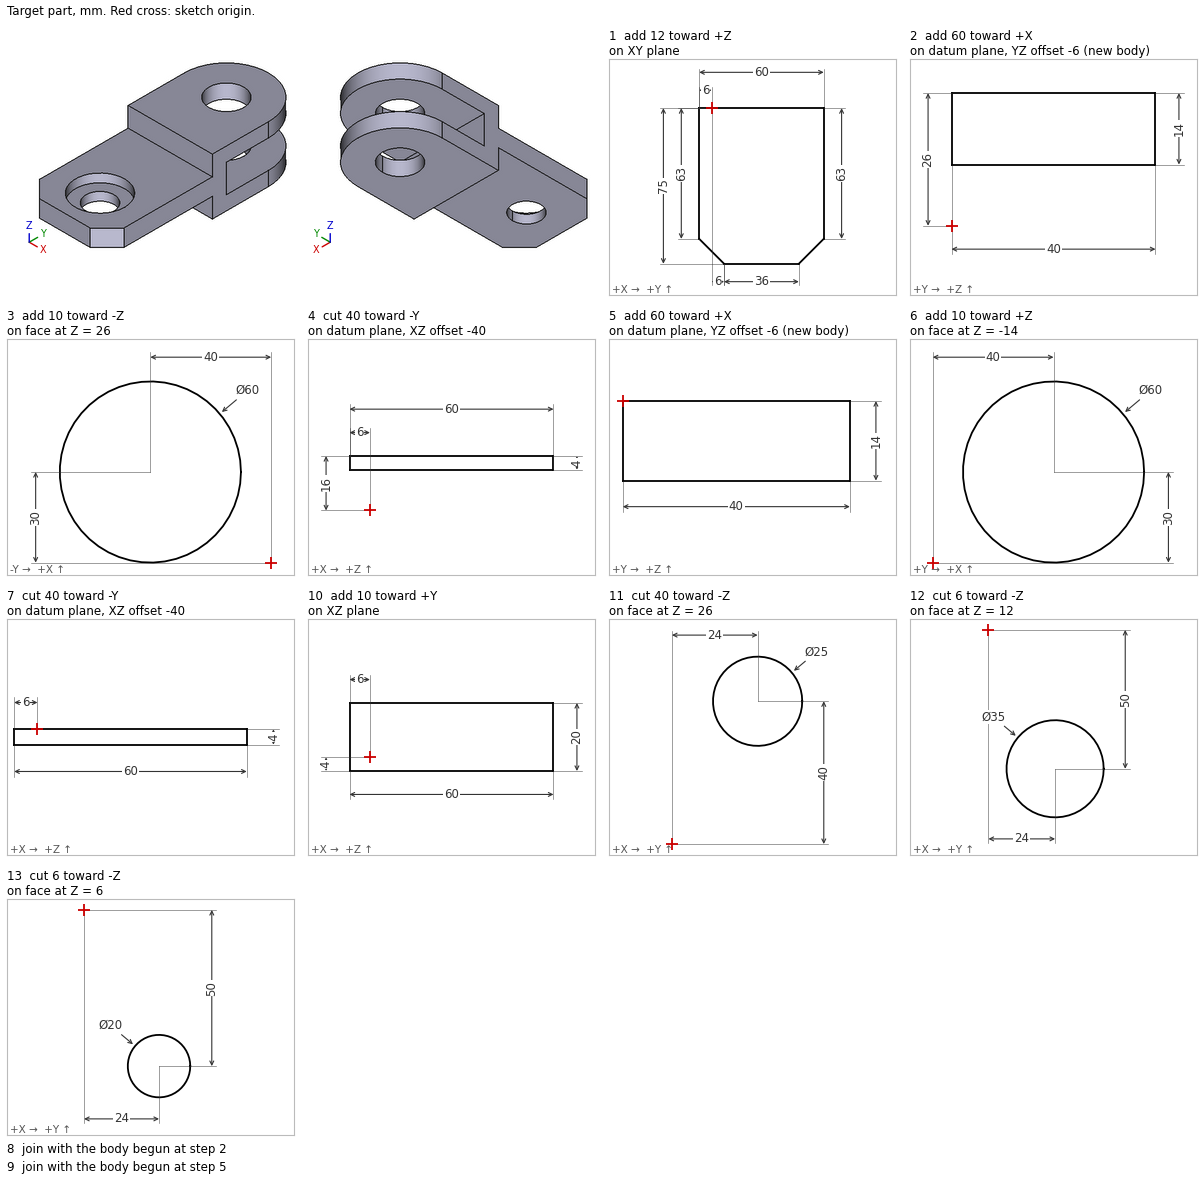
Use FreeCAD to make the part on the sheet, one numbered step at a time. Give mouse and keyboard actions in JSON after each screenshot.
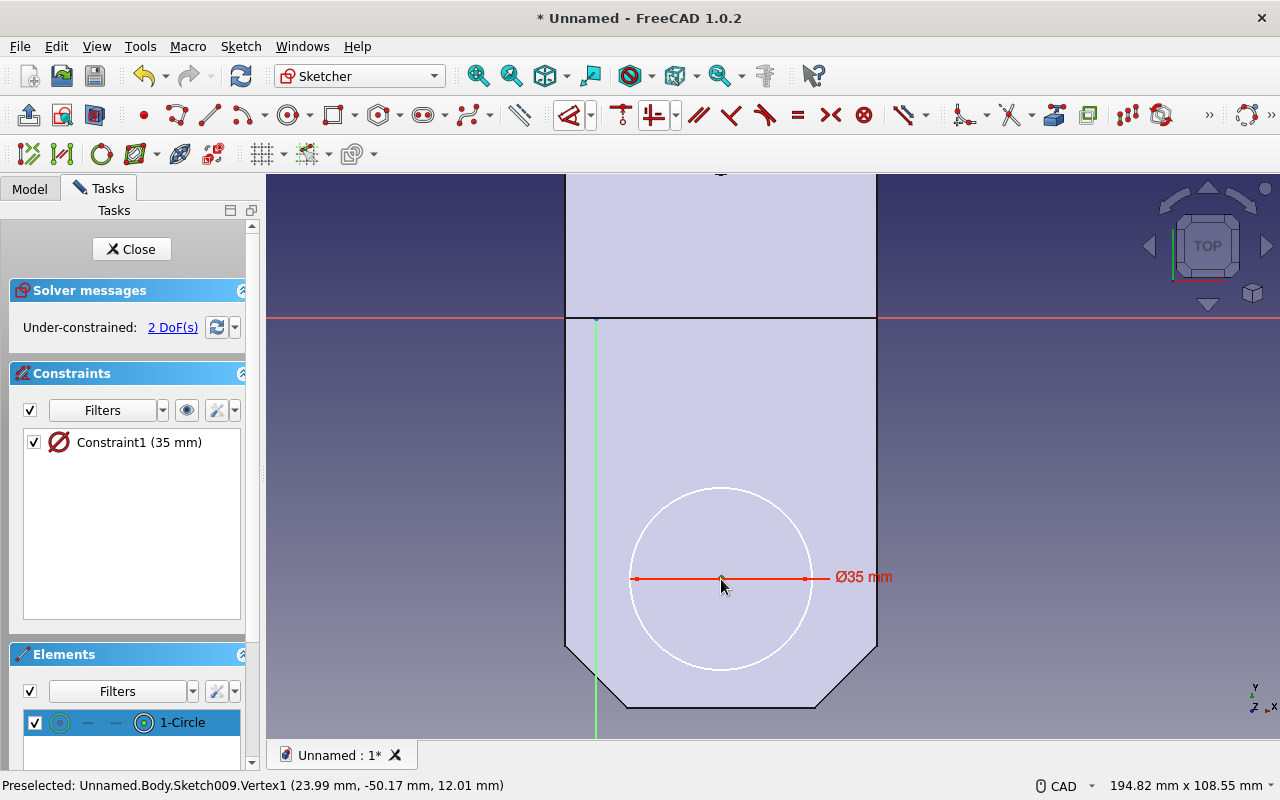
{"action": "left_click", "coordinate": [590, 116]}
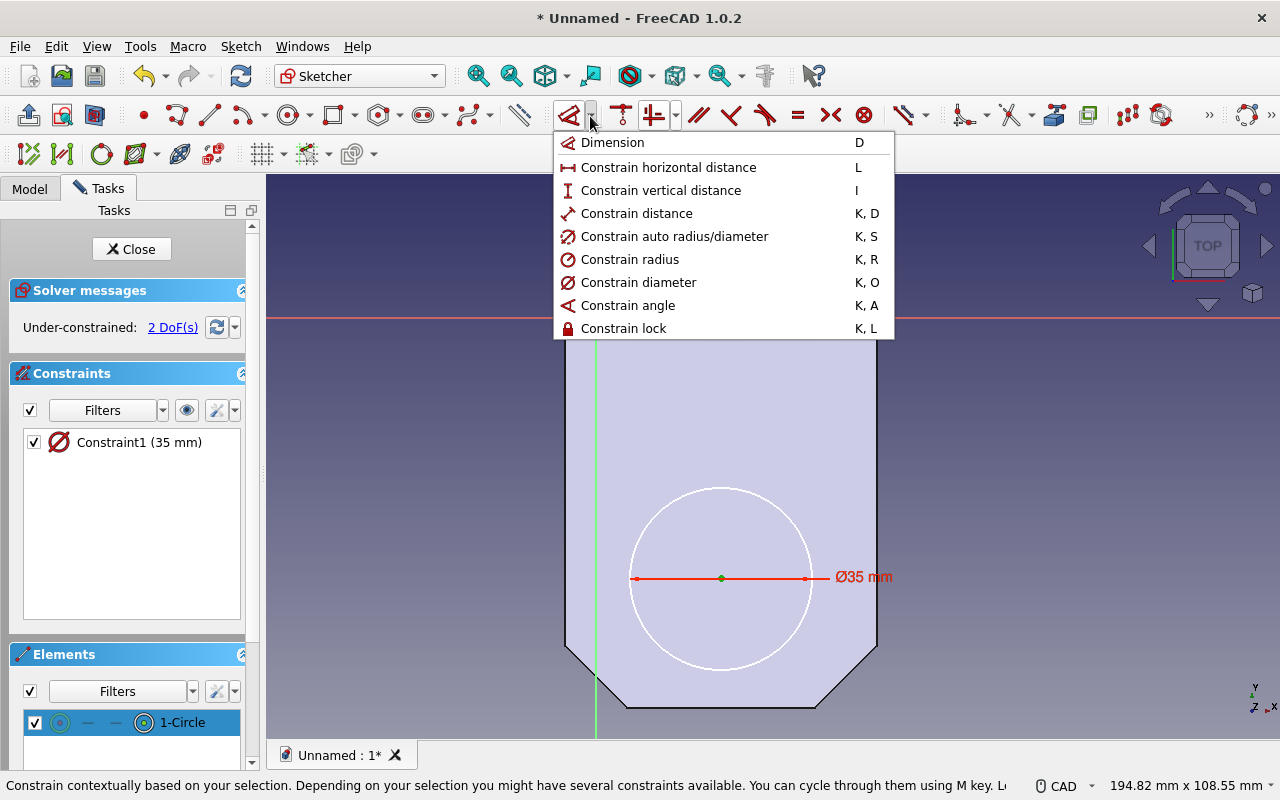
{"action": "left_click", "coordinate": [724, 168]}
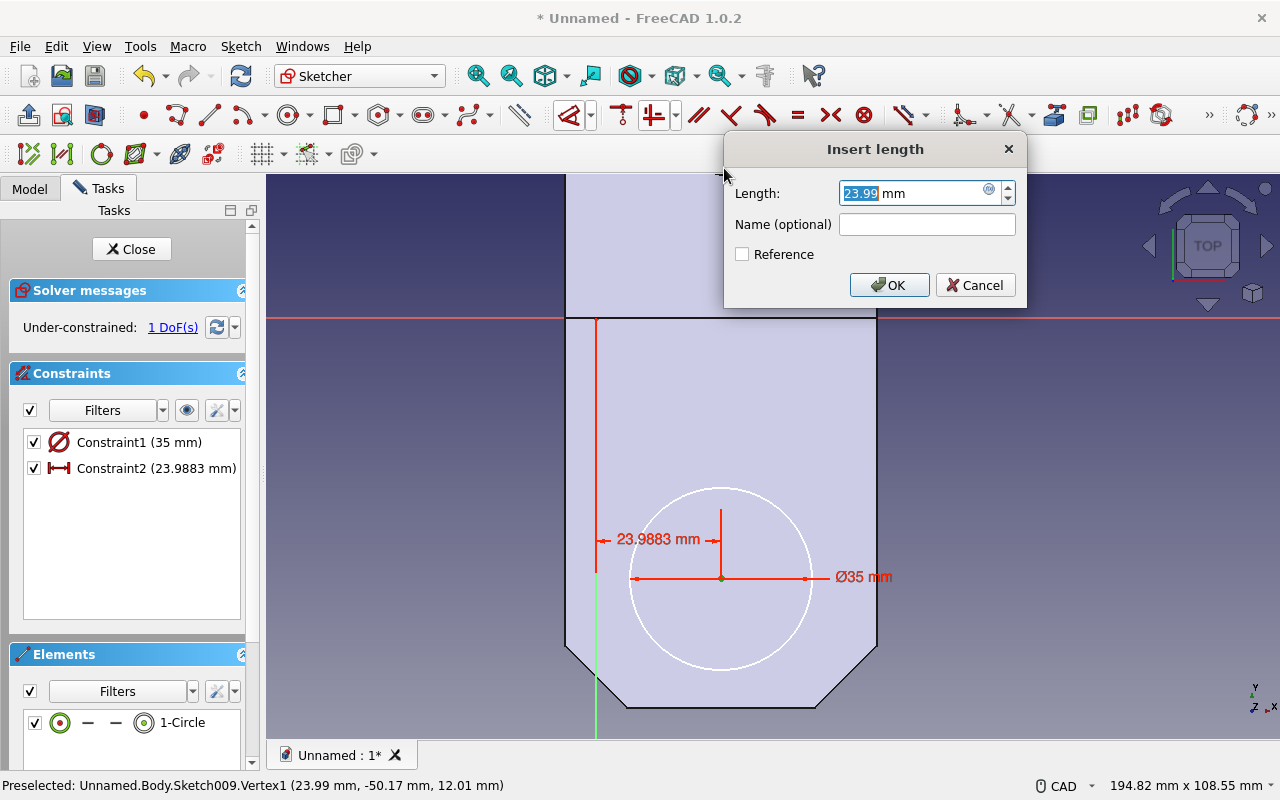
{"action": "type", "text": "24"}
{"action": "key", "text": "Return"}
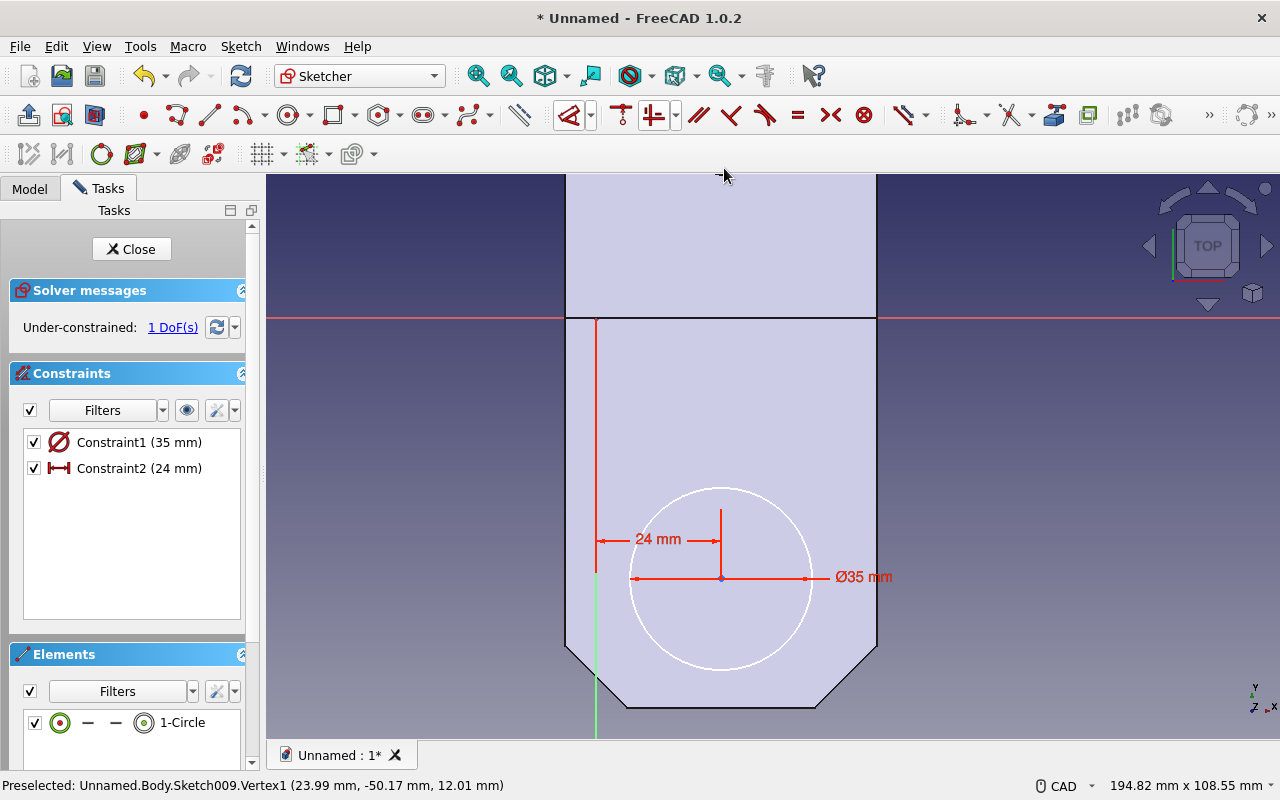
{"action": "left_click", "coordinate": [721, 579]}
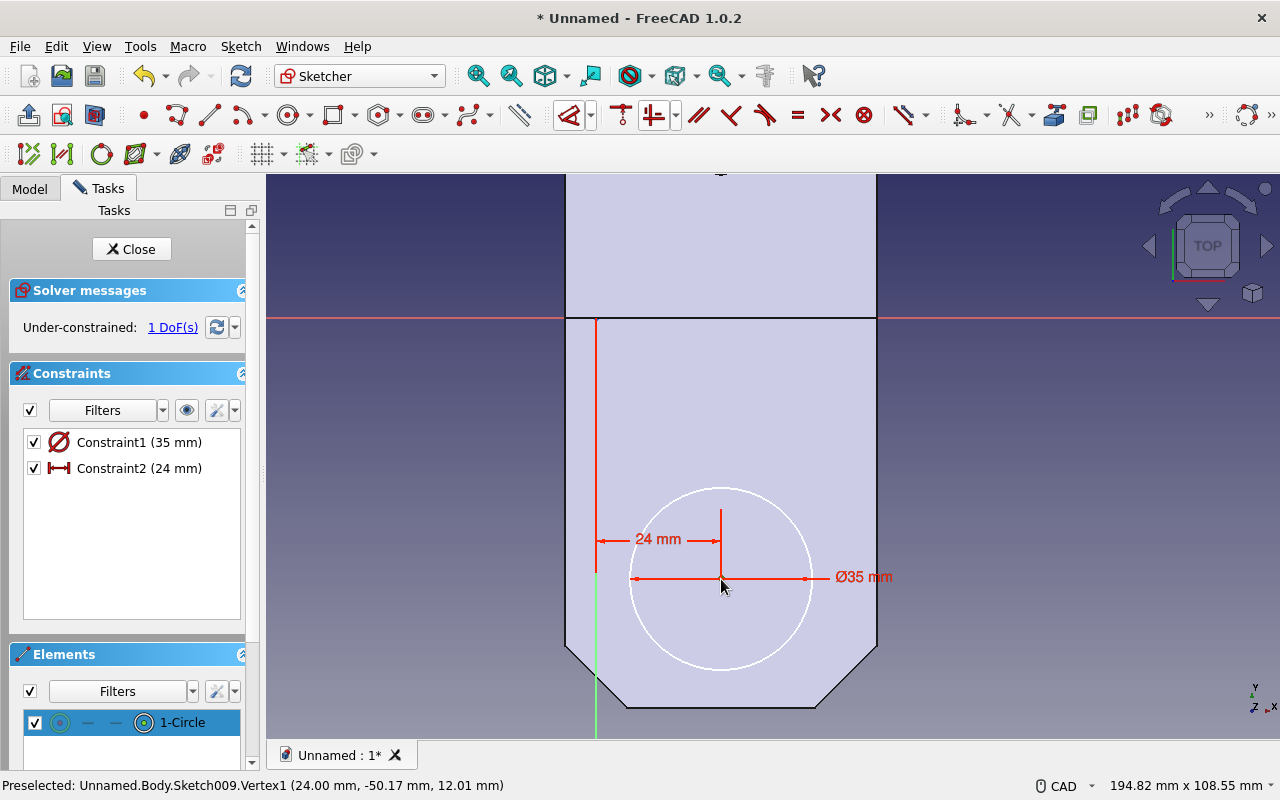
{"action": "left_click", "coordinate": [590, 116]}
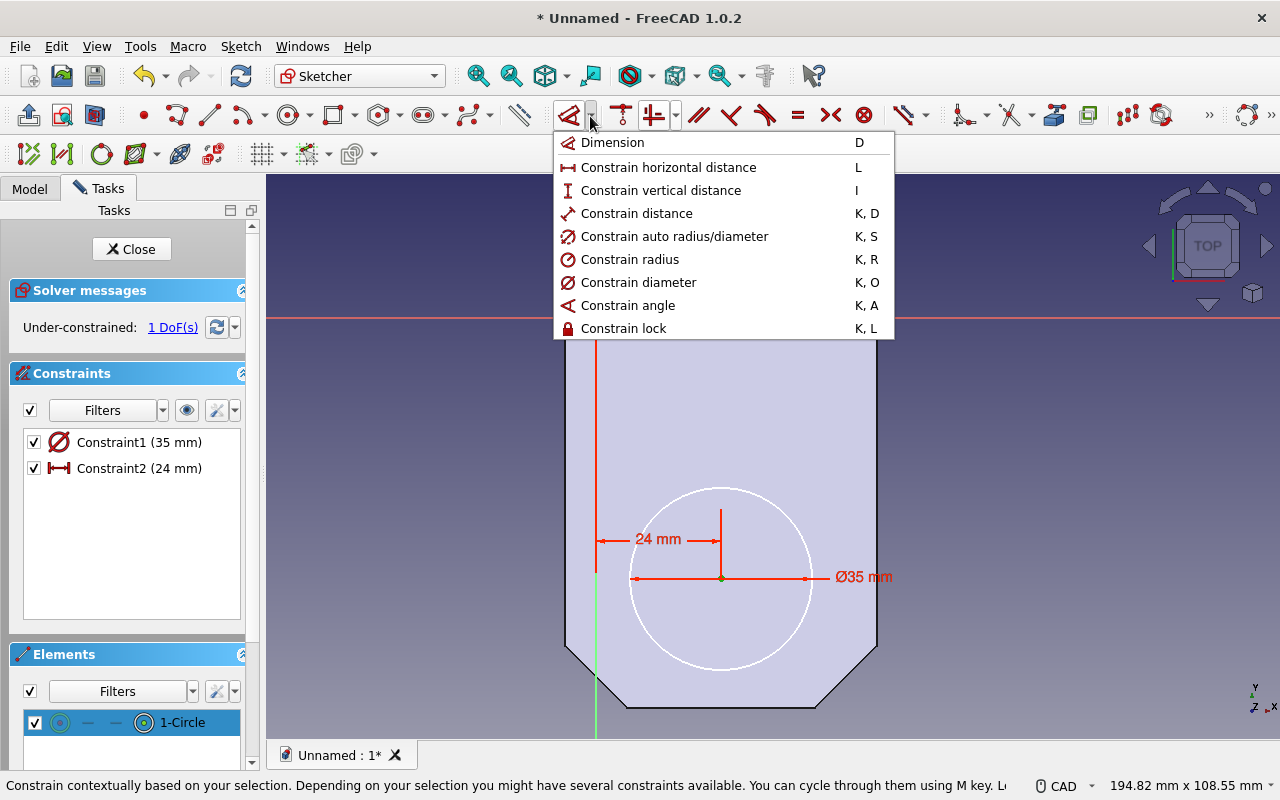
{"action": "left_click", "coordinate": [724, 190]}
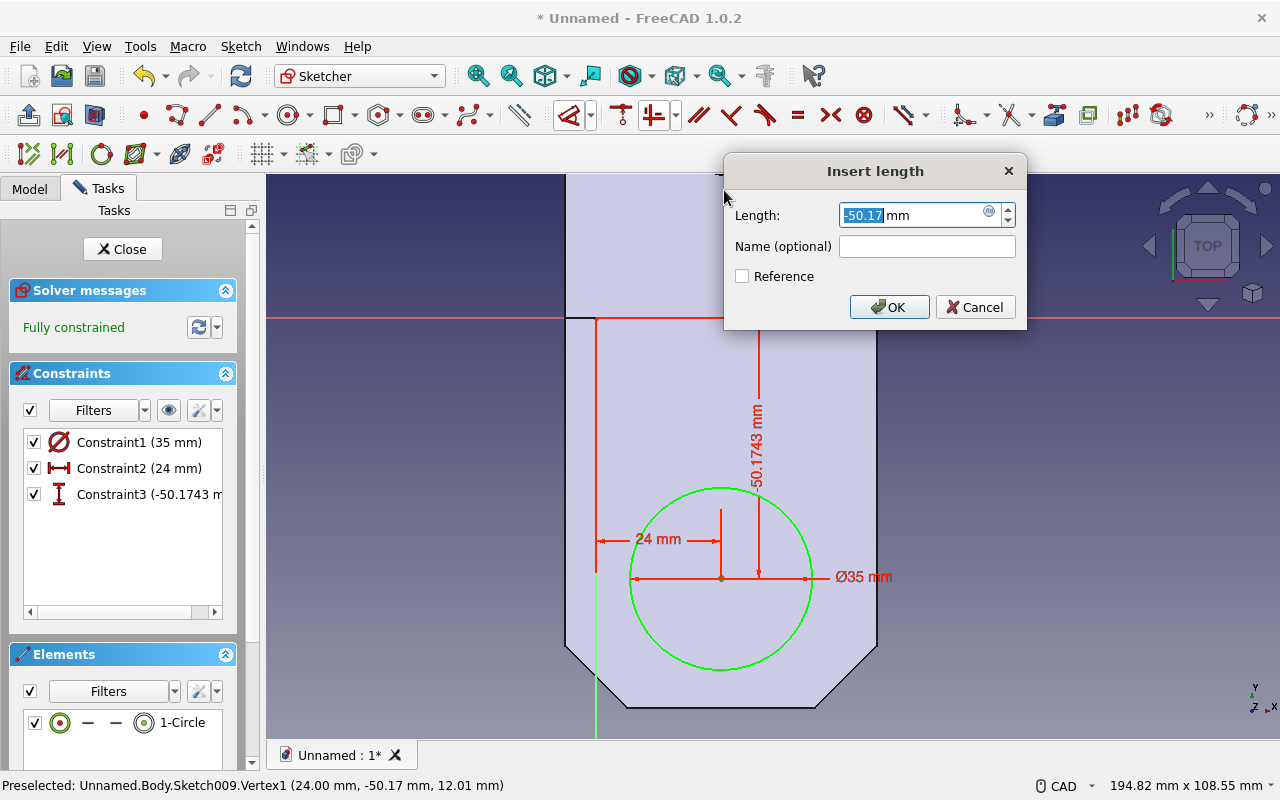
{"action": "type", "text": "-50"}
{"action": "key", "text": "Return"}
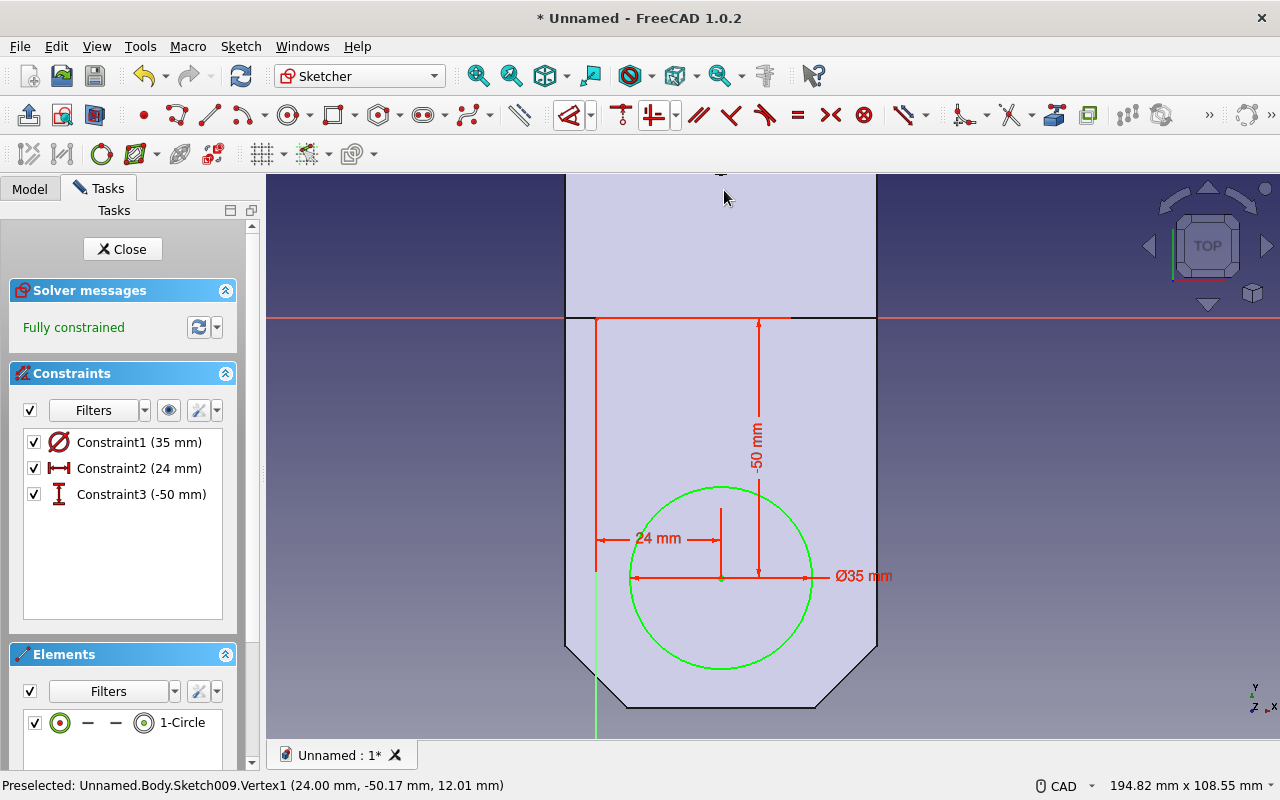
{"action": "left_click", "coordinate": [123, 249]}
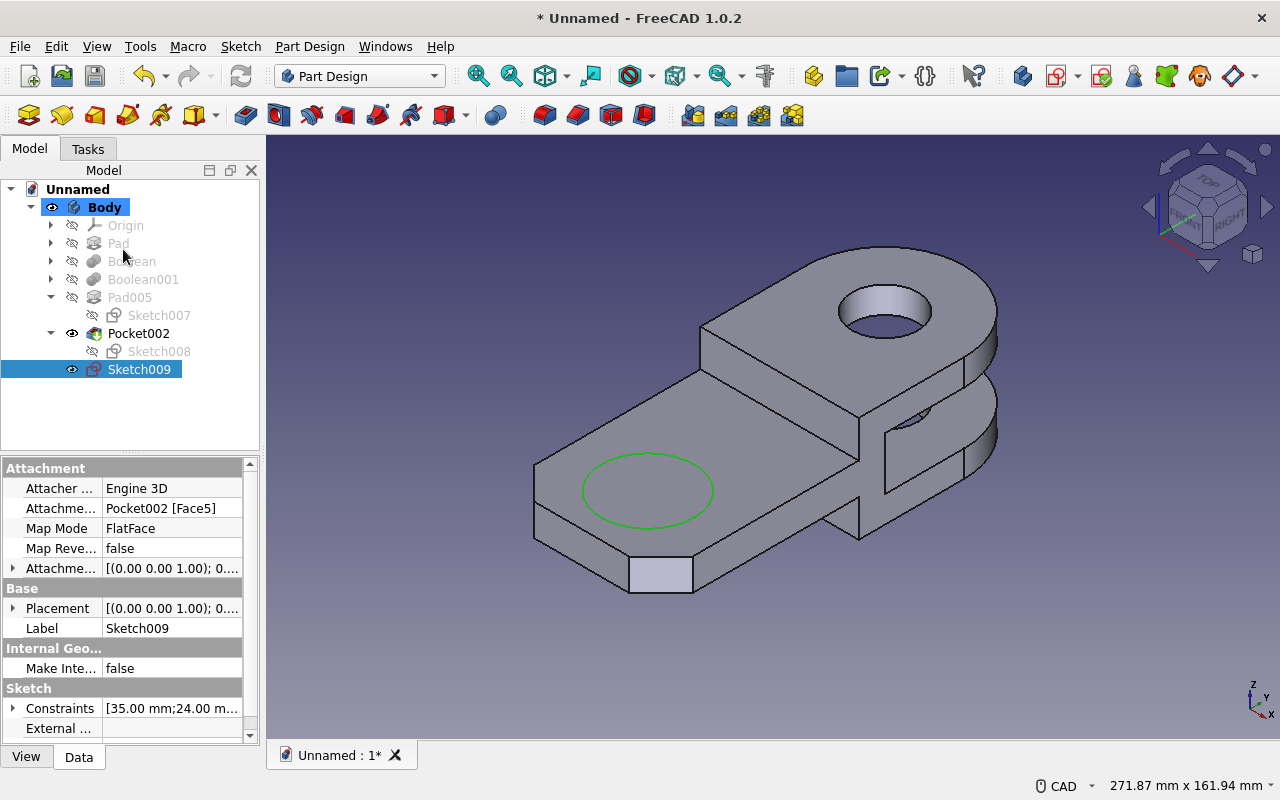
{"action": "left_click", "coordinate": [246, 116]}